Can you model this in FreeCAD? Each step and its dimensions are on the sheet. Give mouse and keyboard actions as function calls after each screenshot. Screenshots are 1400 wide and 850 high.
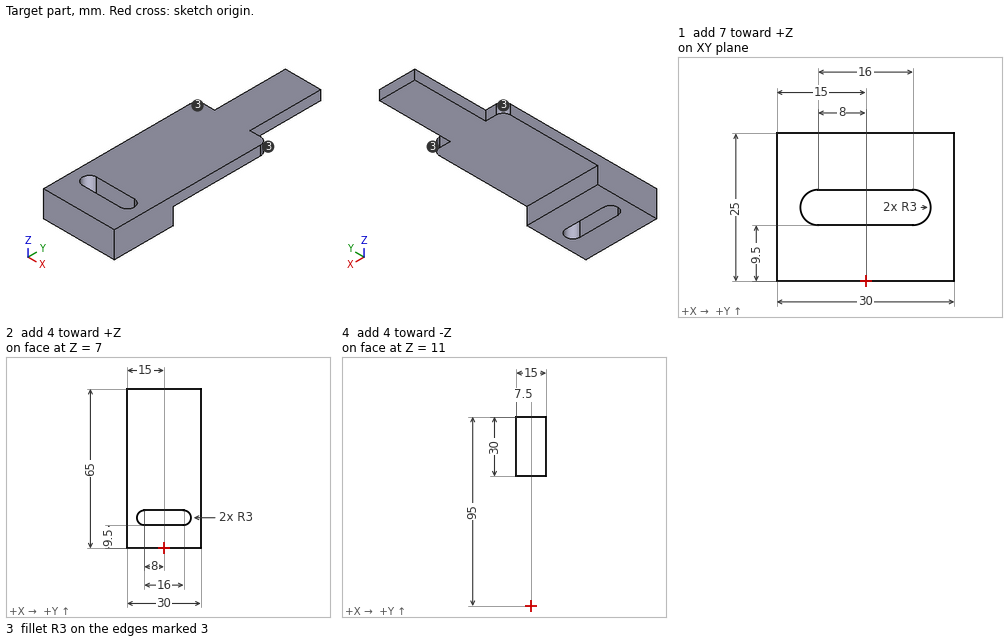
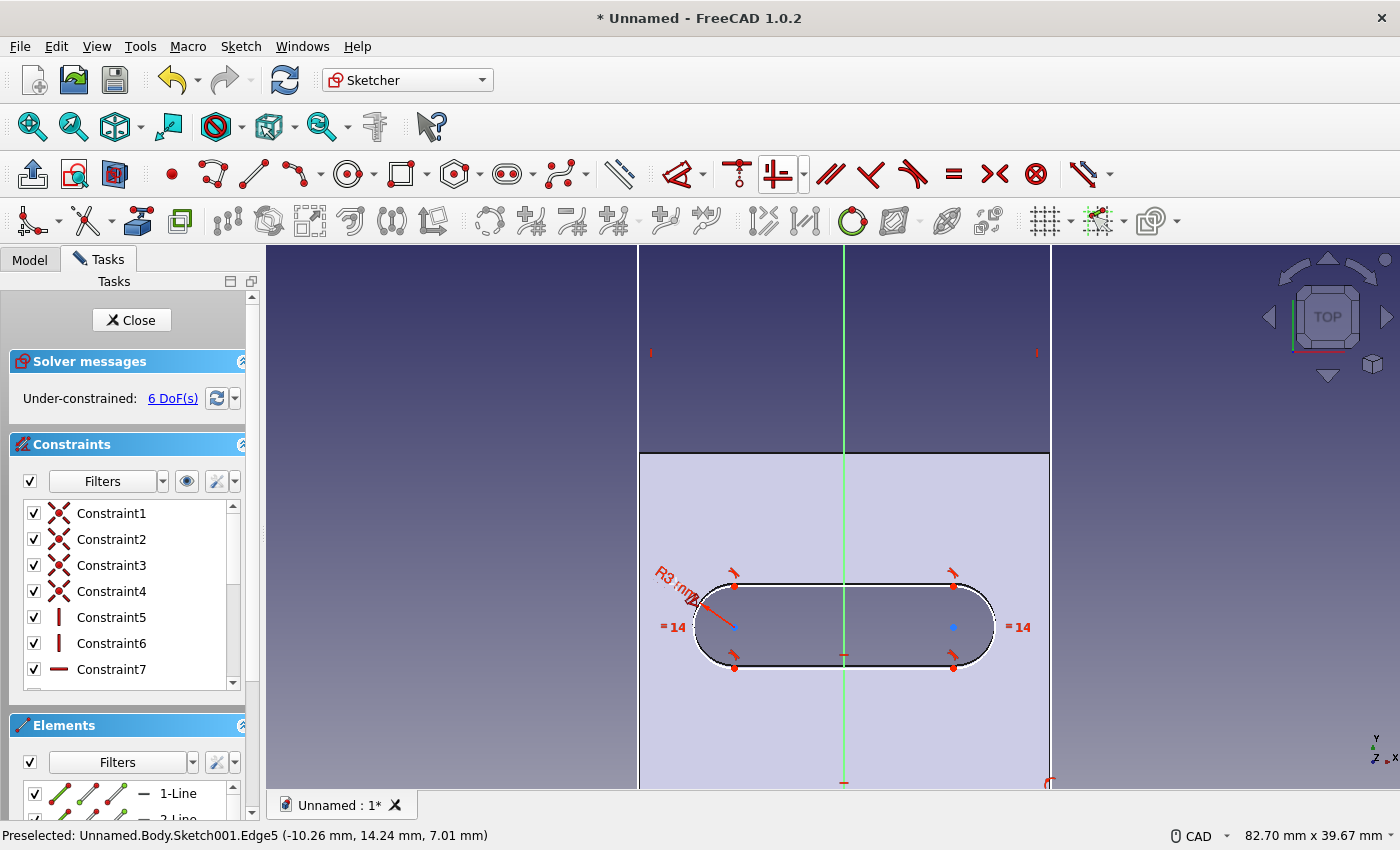
click(638, 530)
click(604, 517)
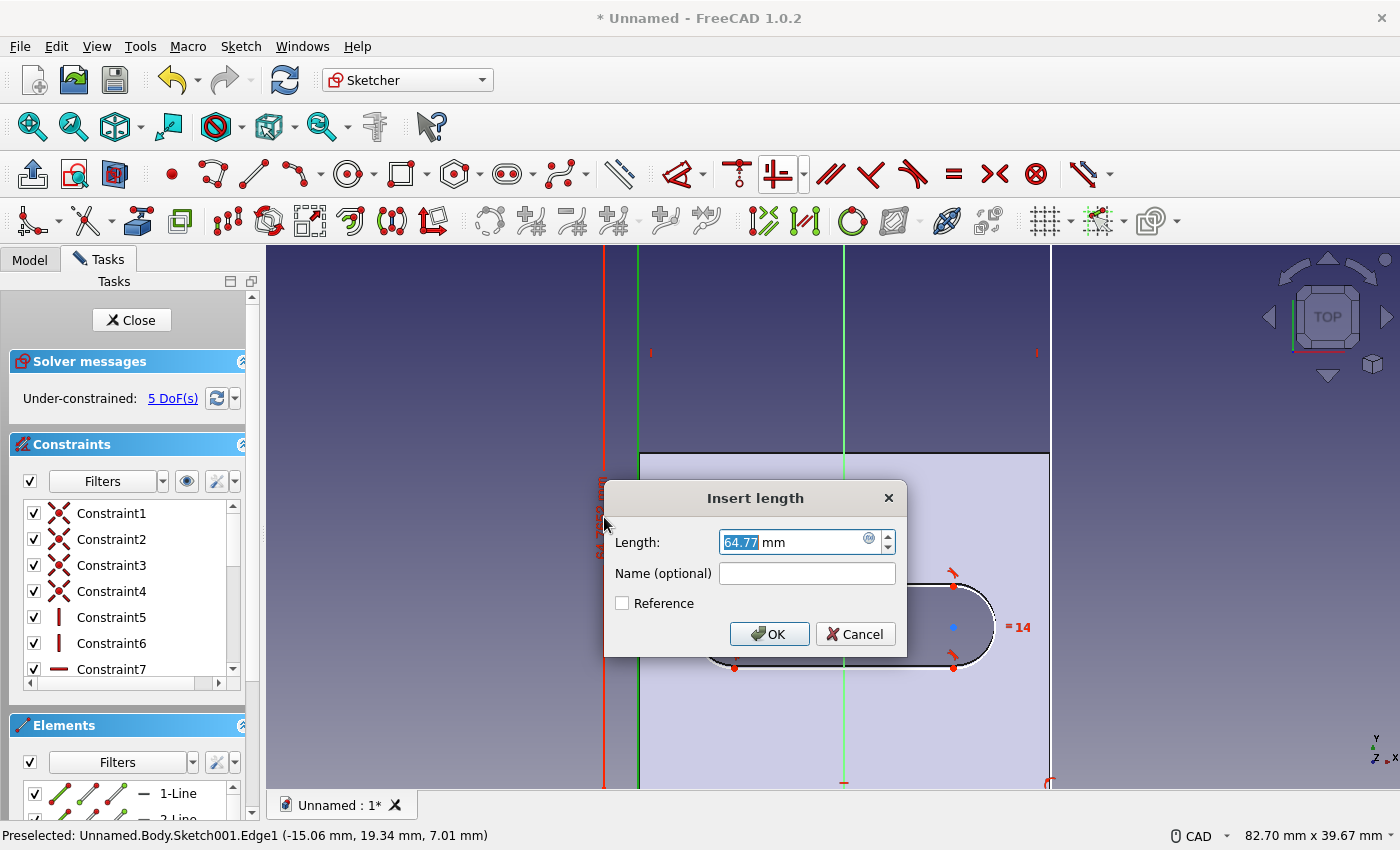
text(65)
key(Return)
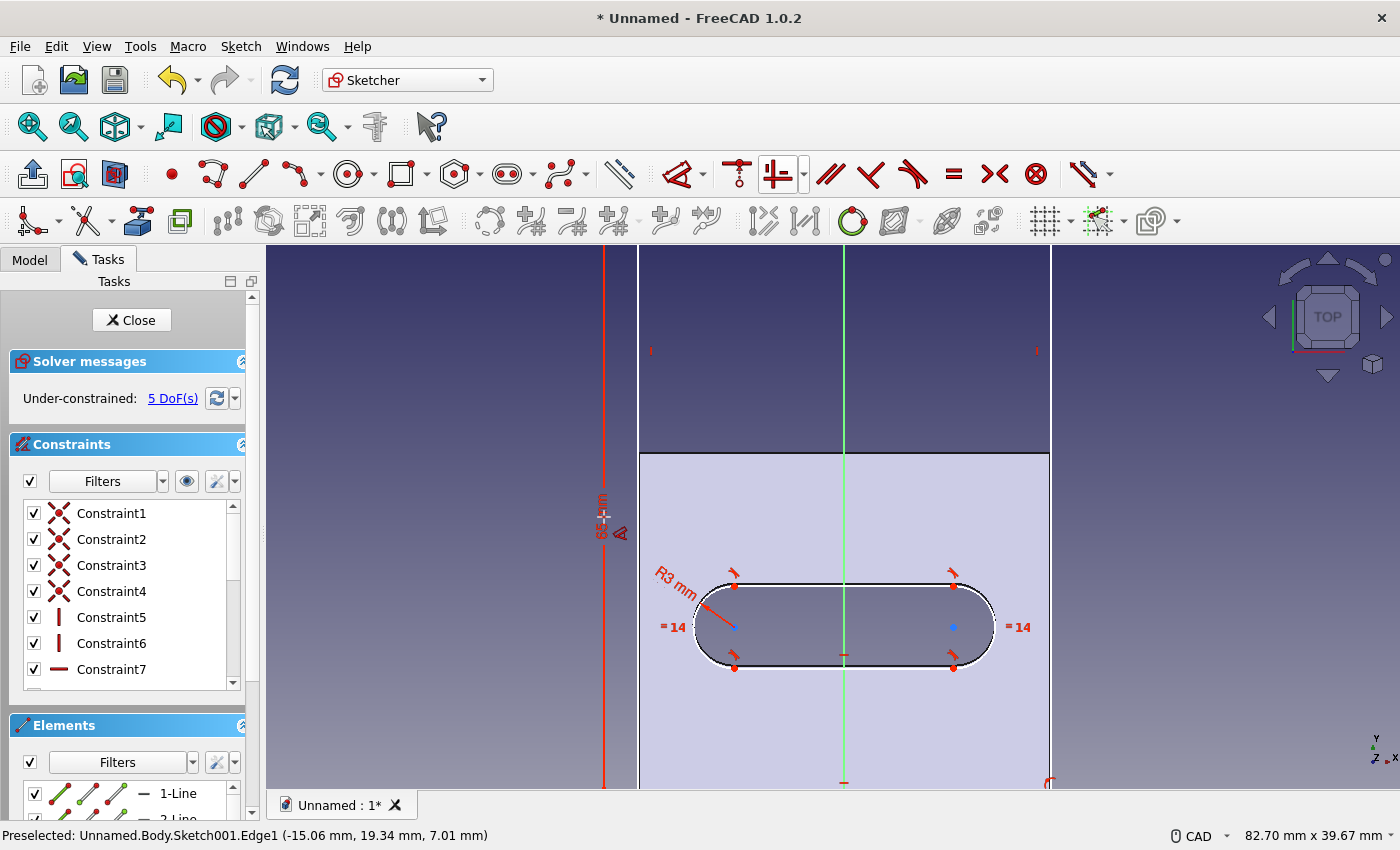
scroll(718, 614, down, 5)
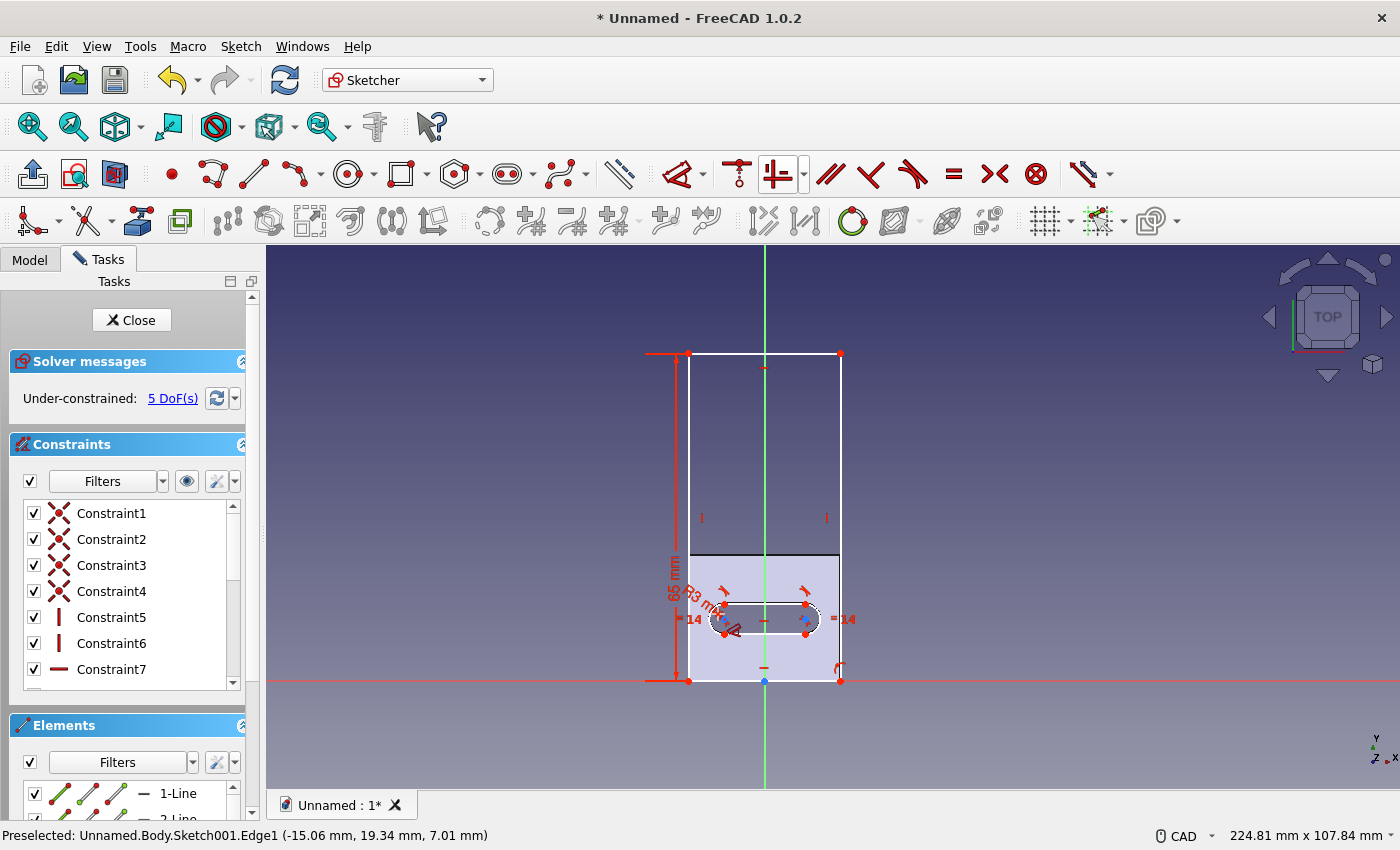
click(734, 681)
click(730, 715)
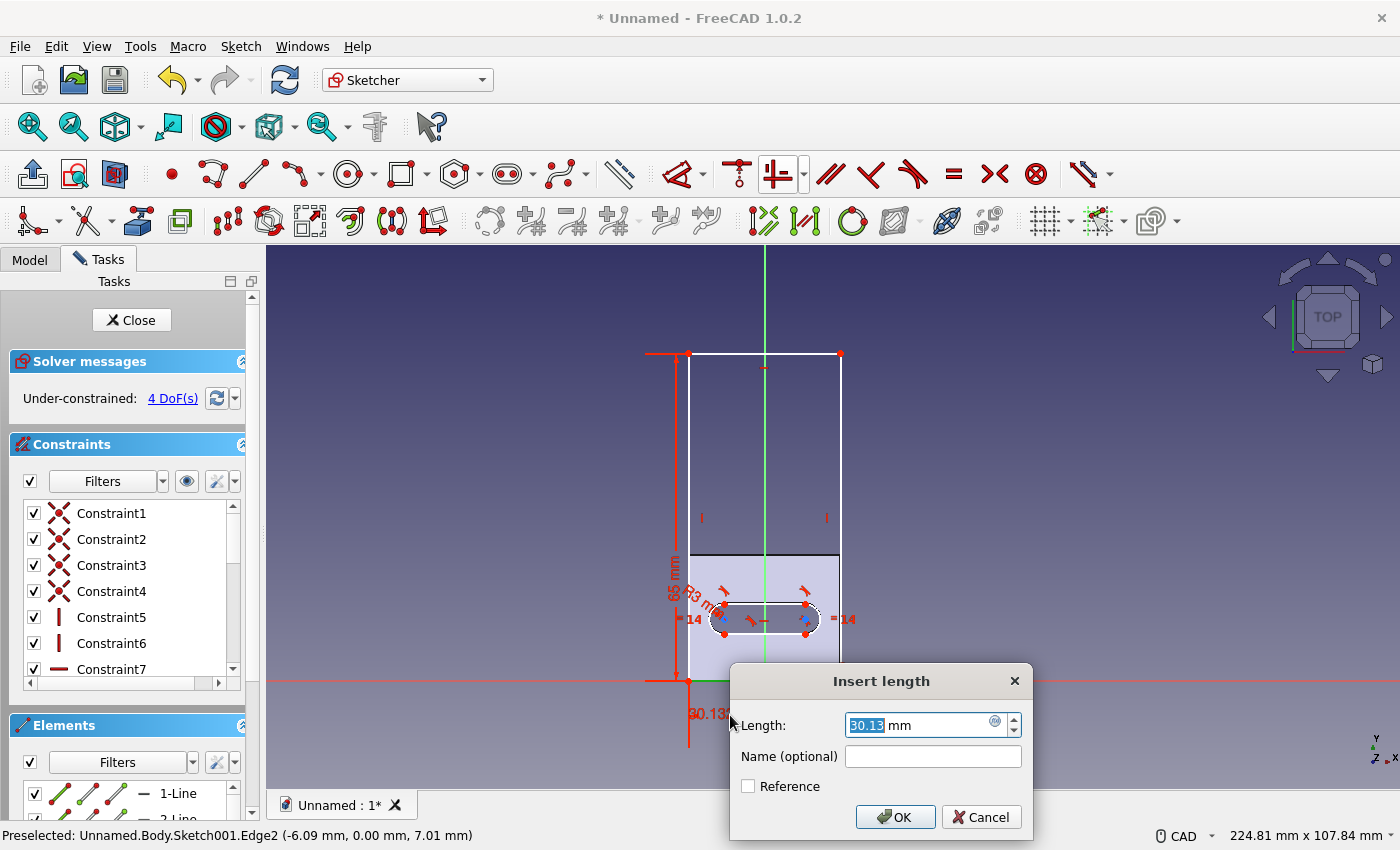
text(30)
key(Return)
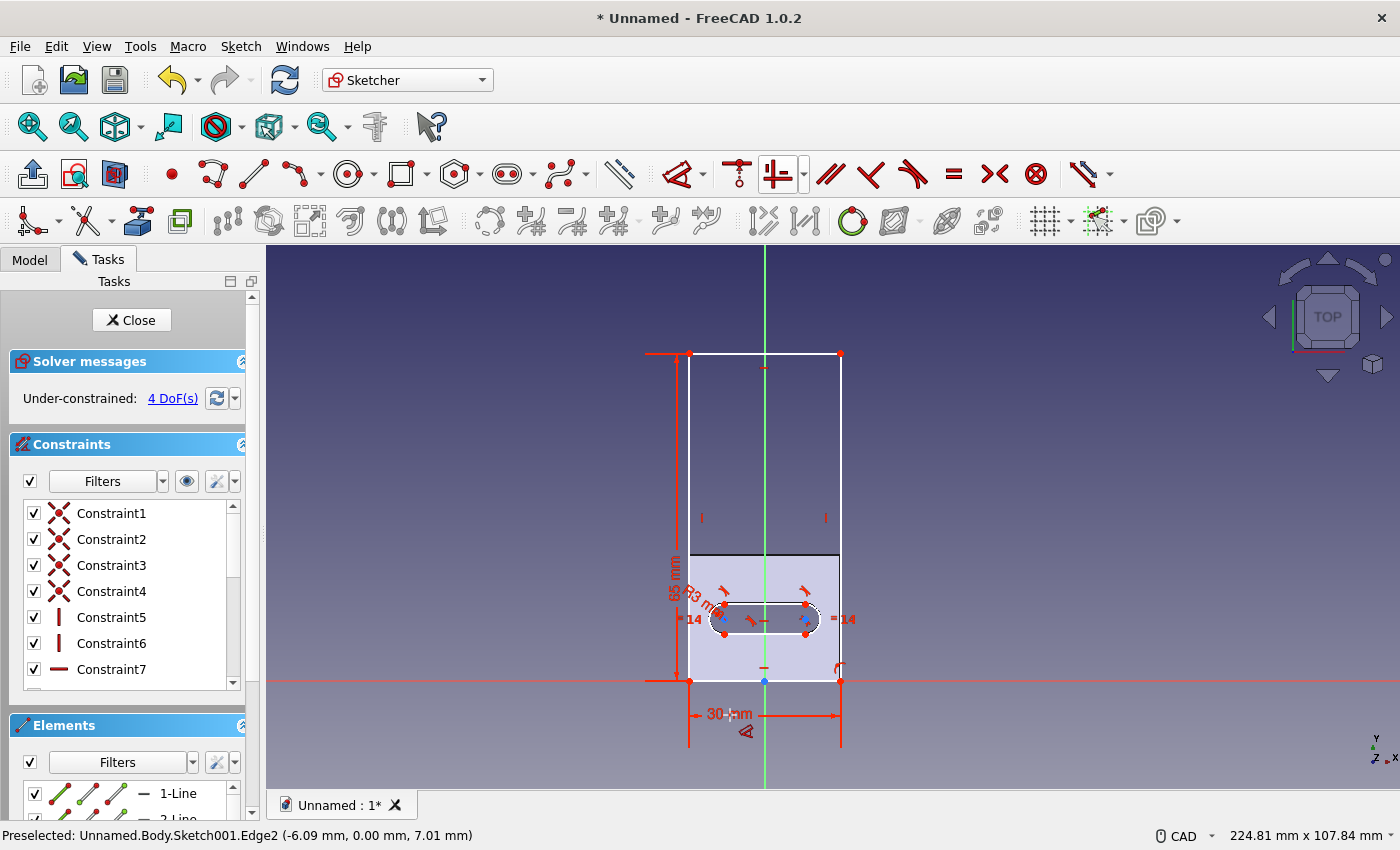
click(749, 604)
click(783, 570)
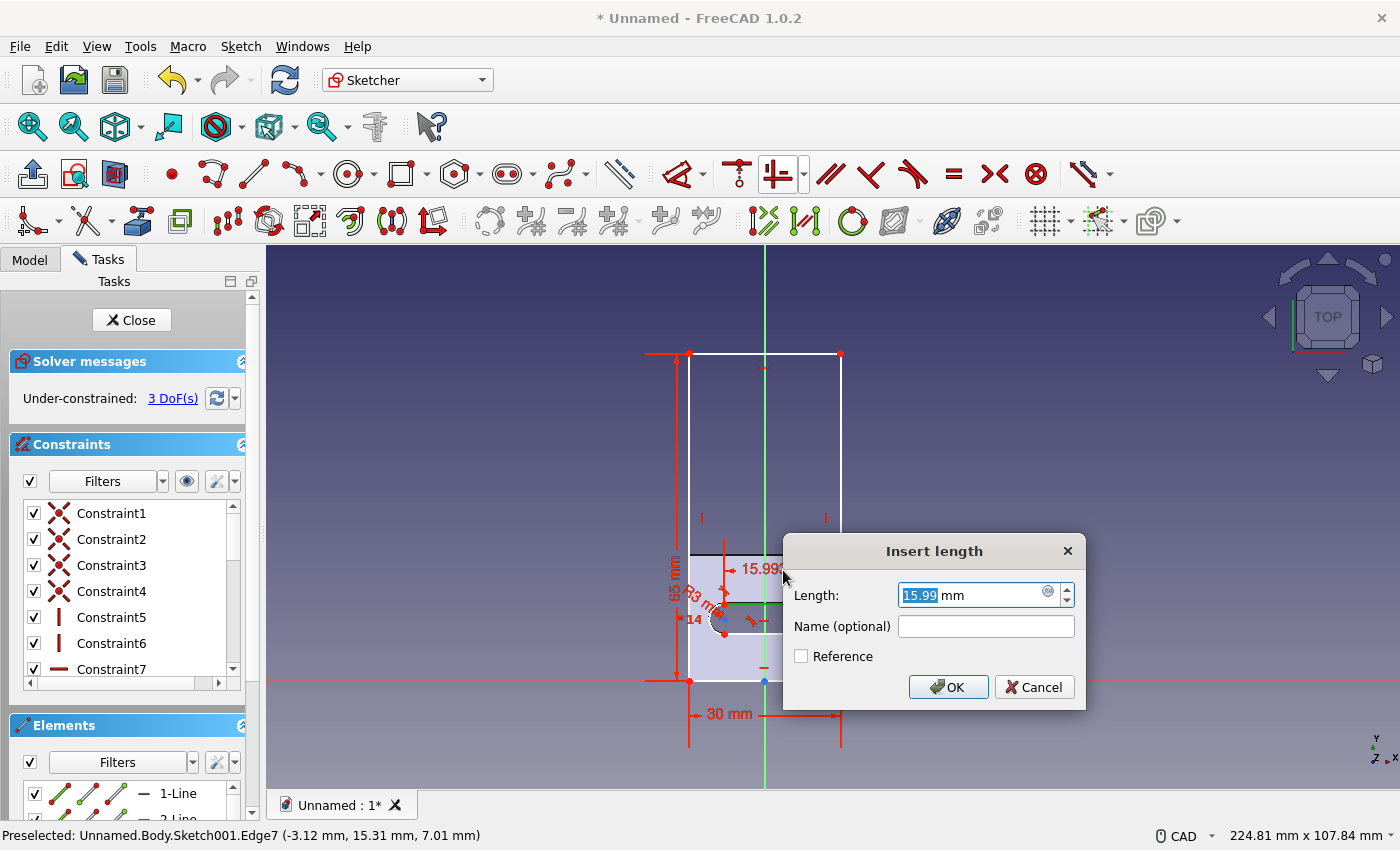
text(16)
key(Return)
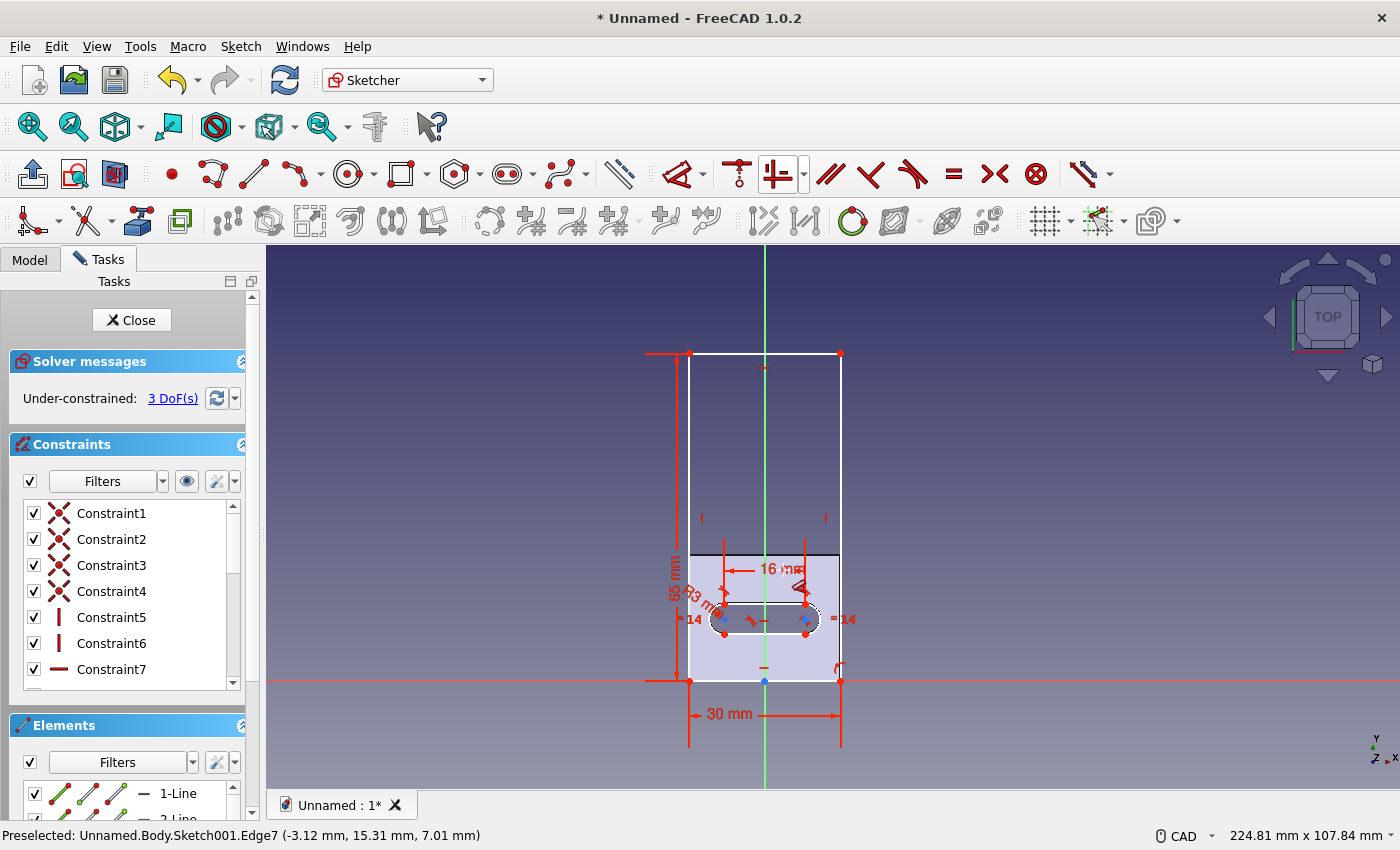
click(724, 604)
click(745, 739)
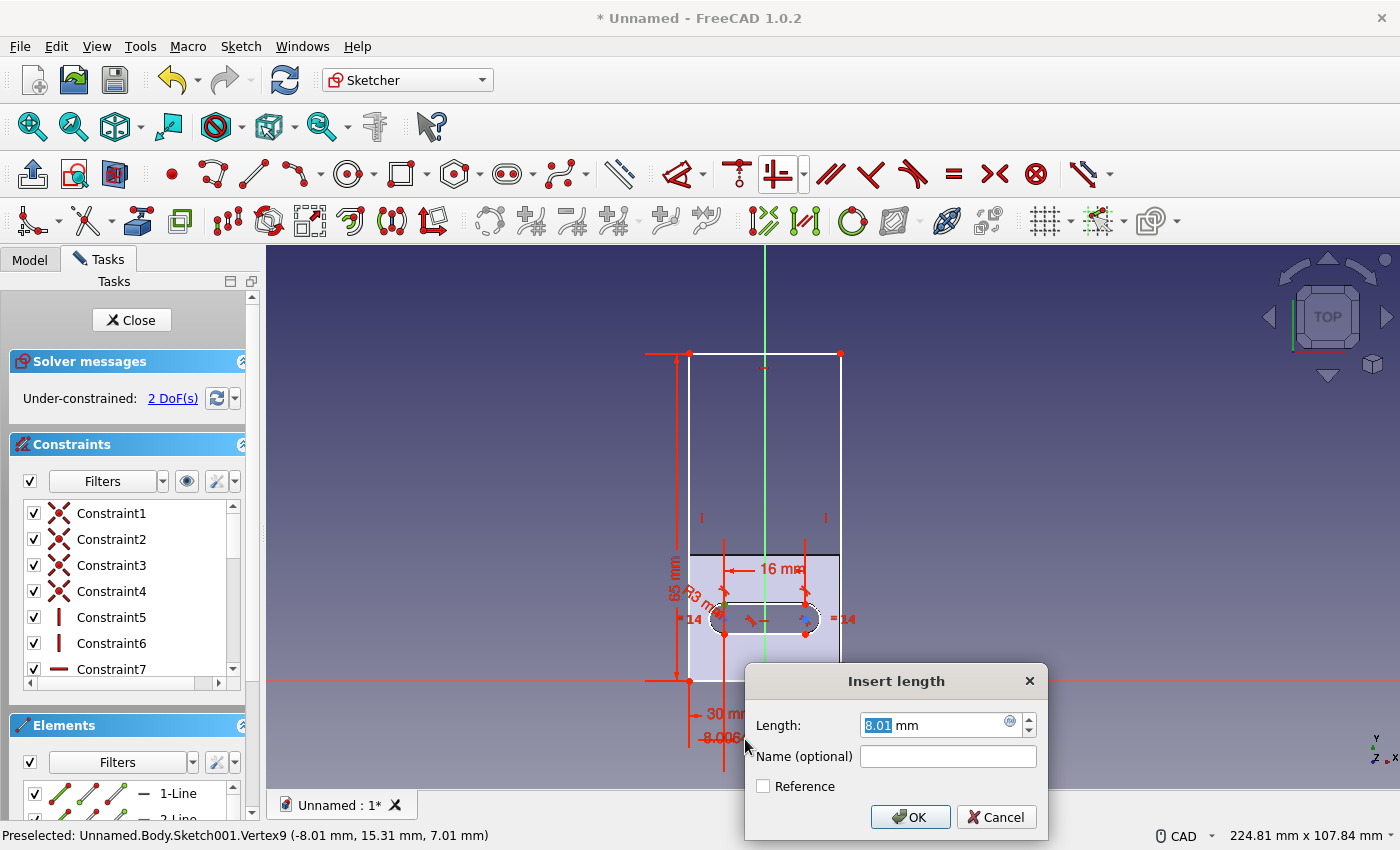
text(8)
key(Return)